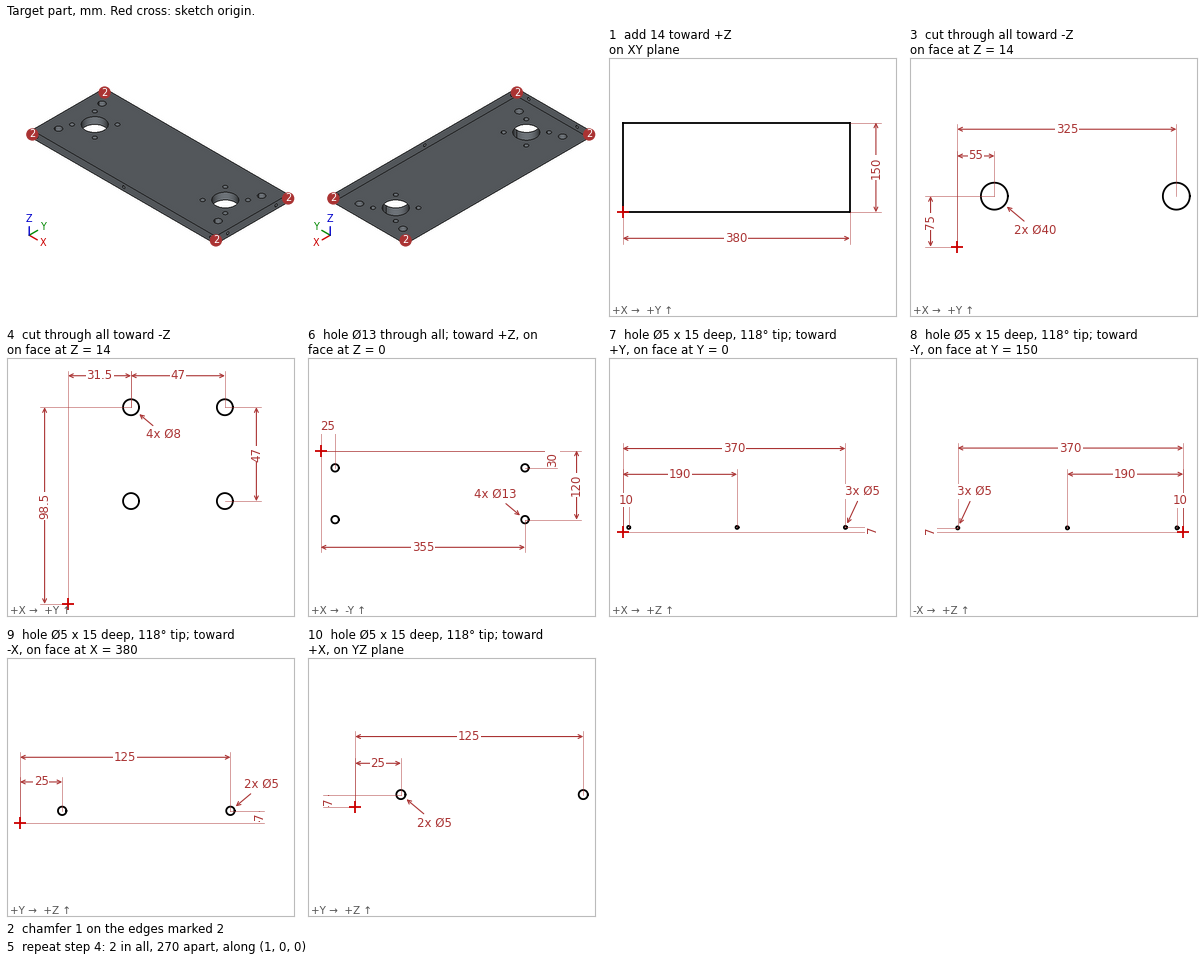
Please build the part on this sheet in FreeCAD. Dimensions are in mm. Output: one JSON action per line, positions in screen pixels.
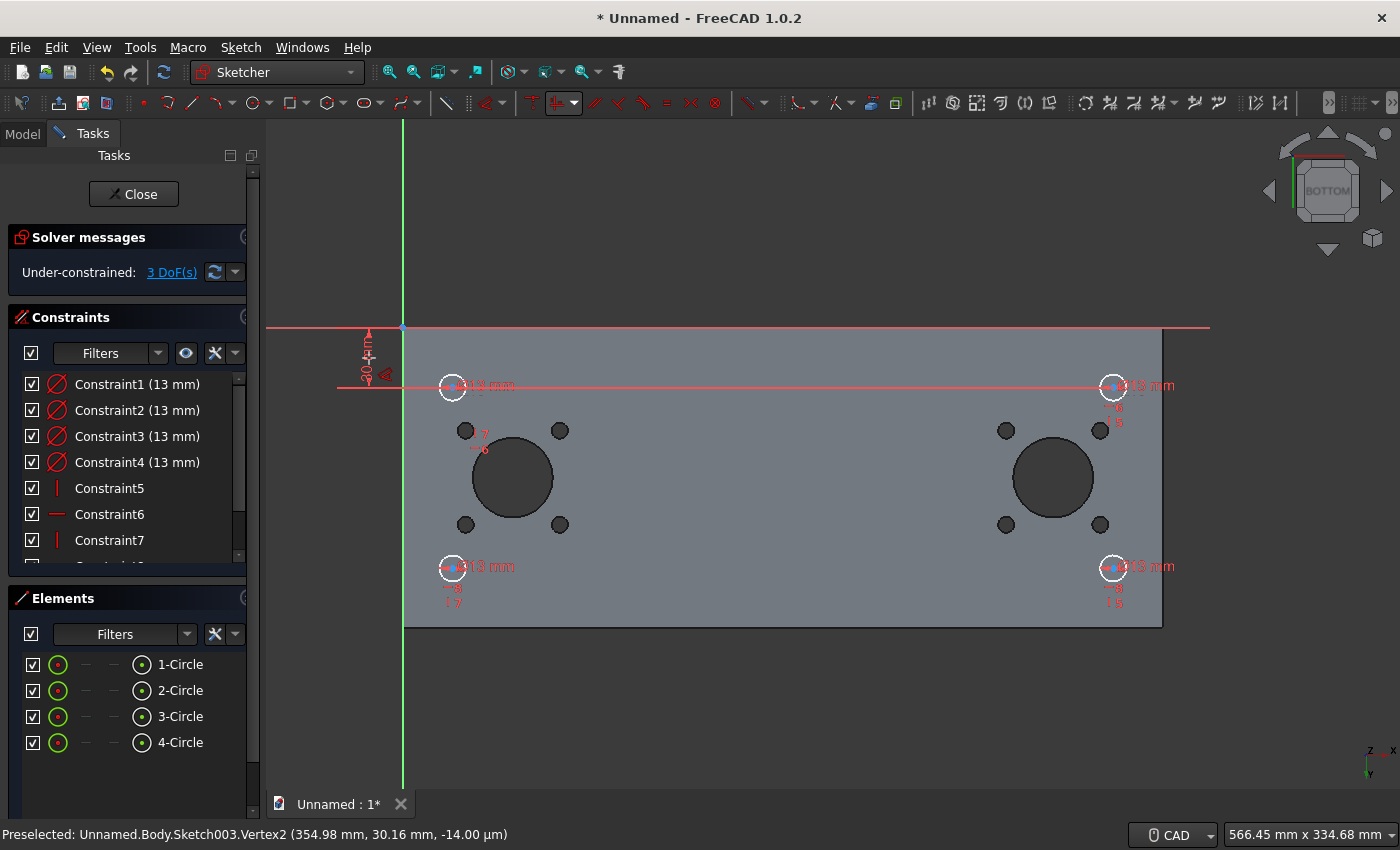
{"action": "left_click", "coordinate": [453, 388]}
{"action": "left_click", "coordinate": [428, 294]}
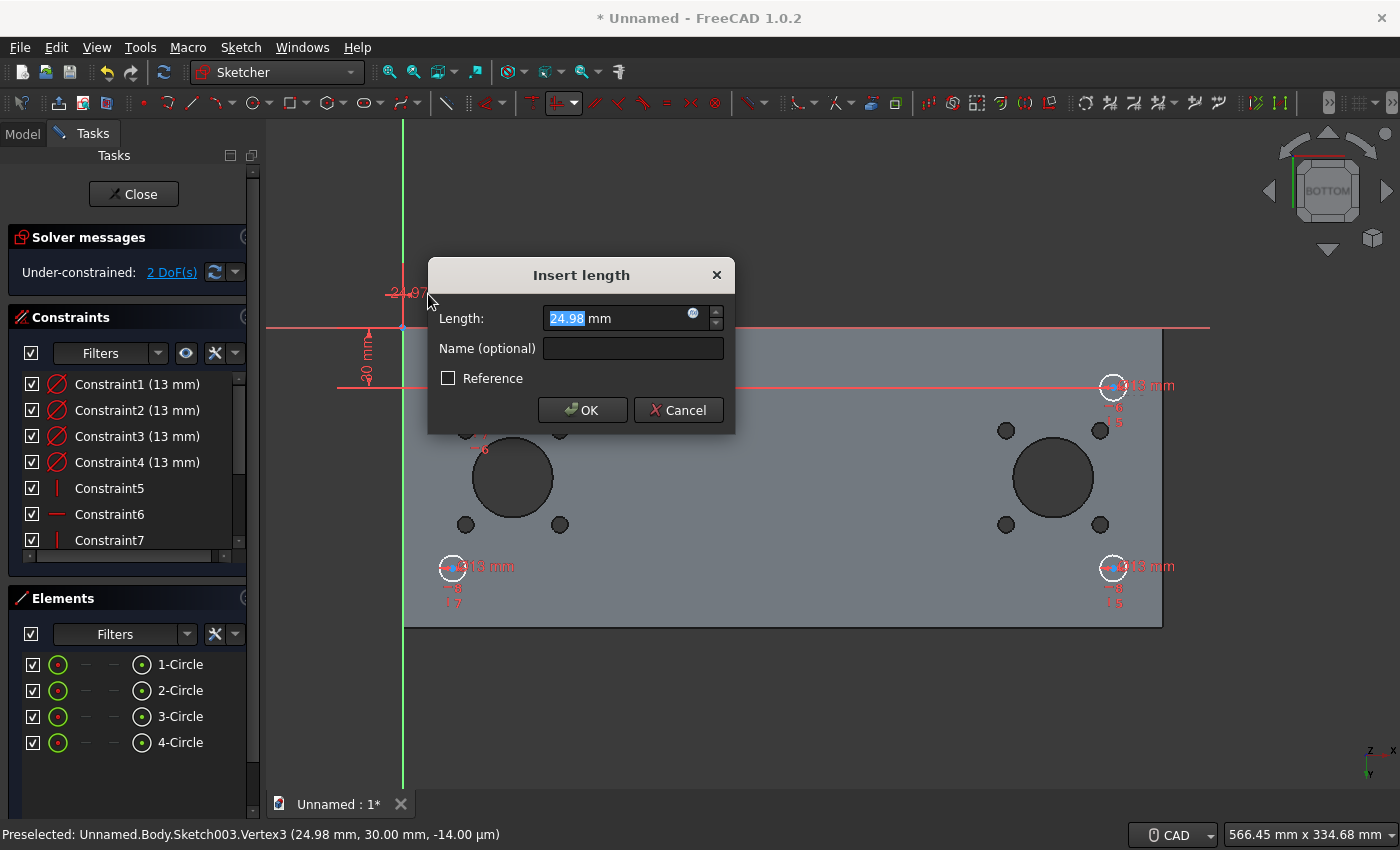
{"action": "type", "text": "25"}
{"action": "key", "text": "Return"}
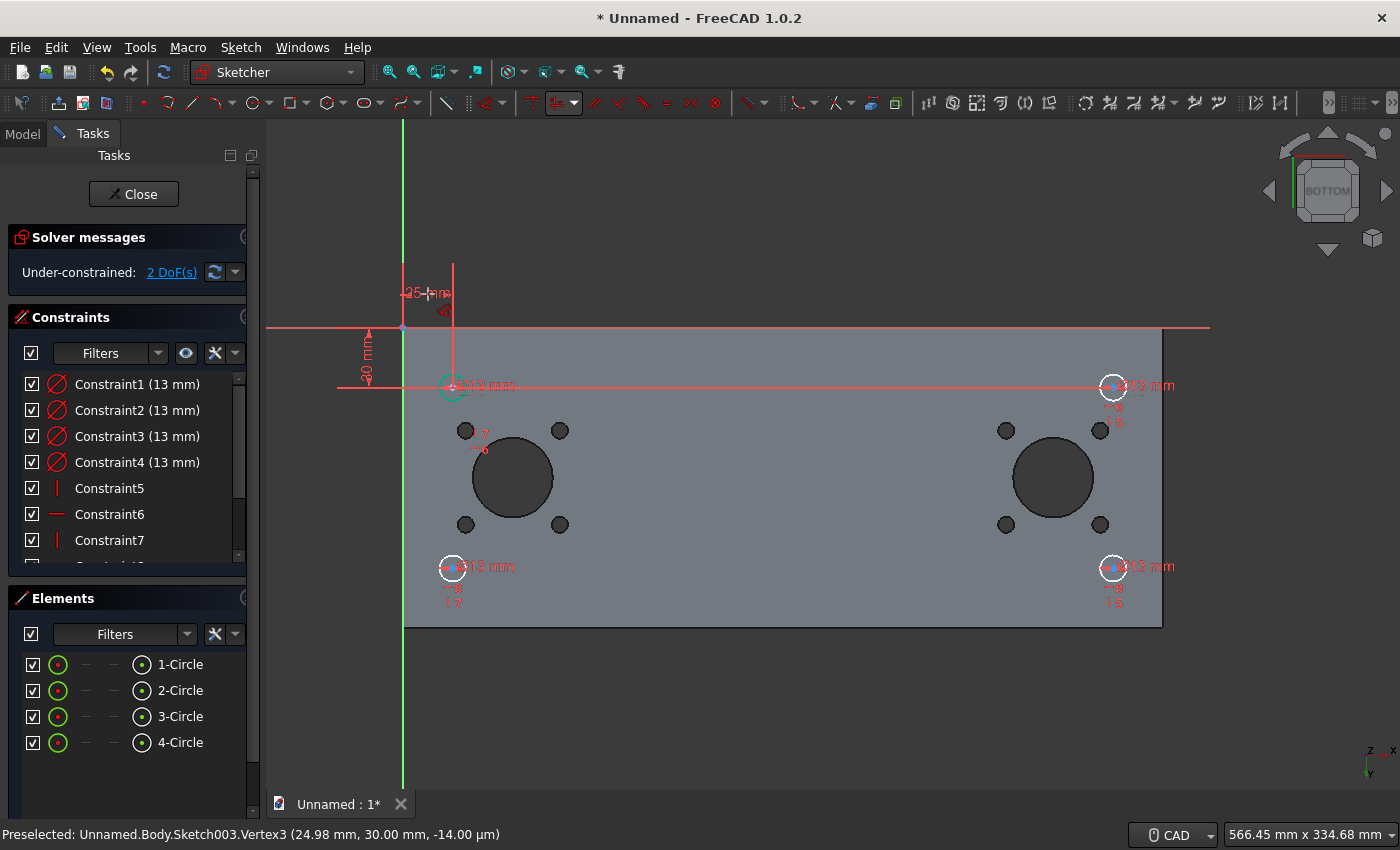
{"action": "left_click", "coordinate": [1113, 568]}
{"action": "left_click", "coordinate": [758, 294]}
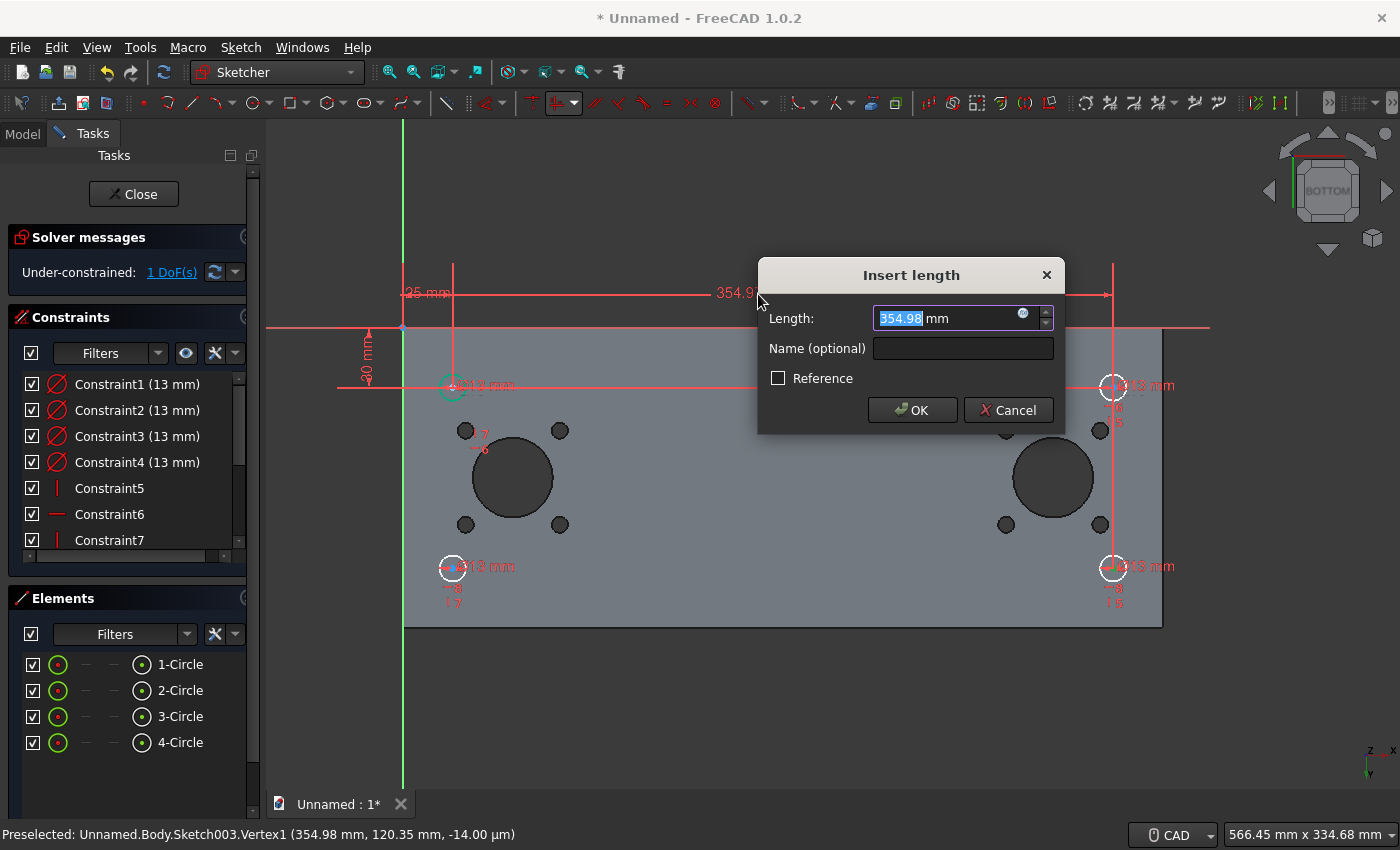
{"action": "type", "text": "355"}
{"action": "key", "text": "Return"}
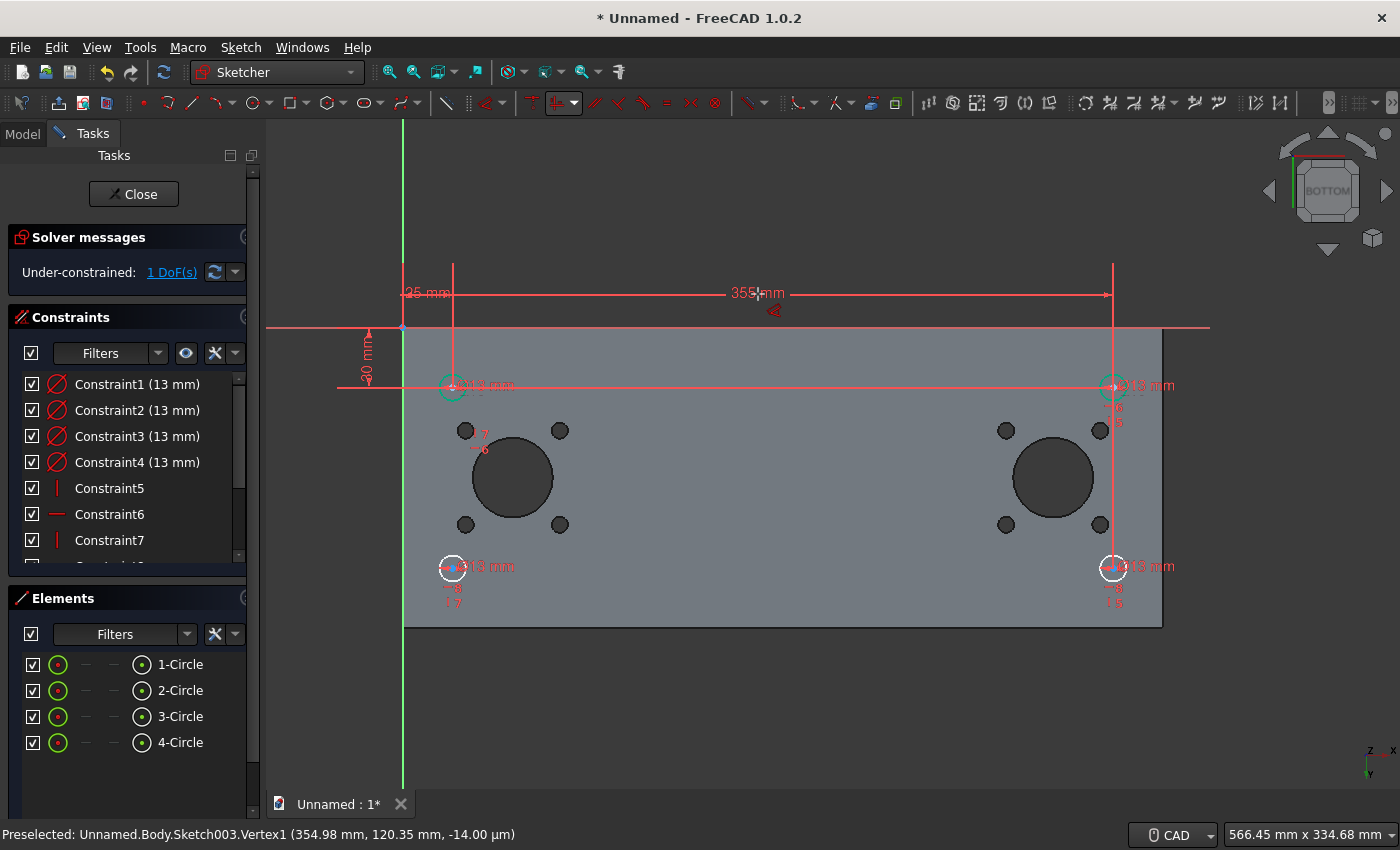
{"action": "left_click", "coordinate": [1113, 568]}
{"action": "left_click", "coordinate": [369, 448]}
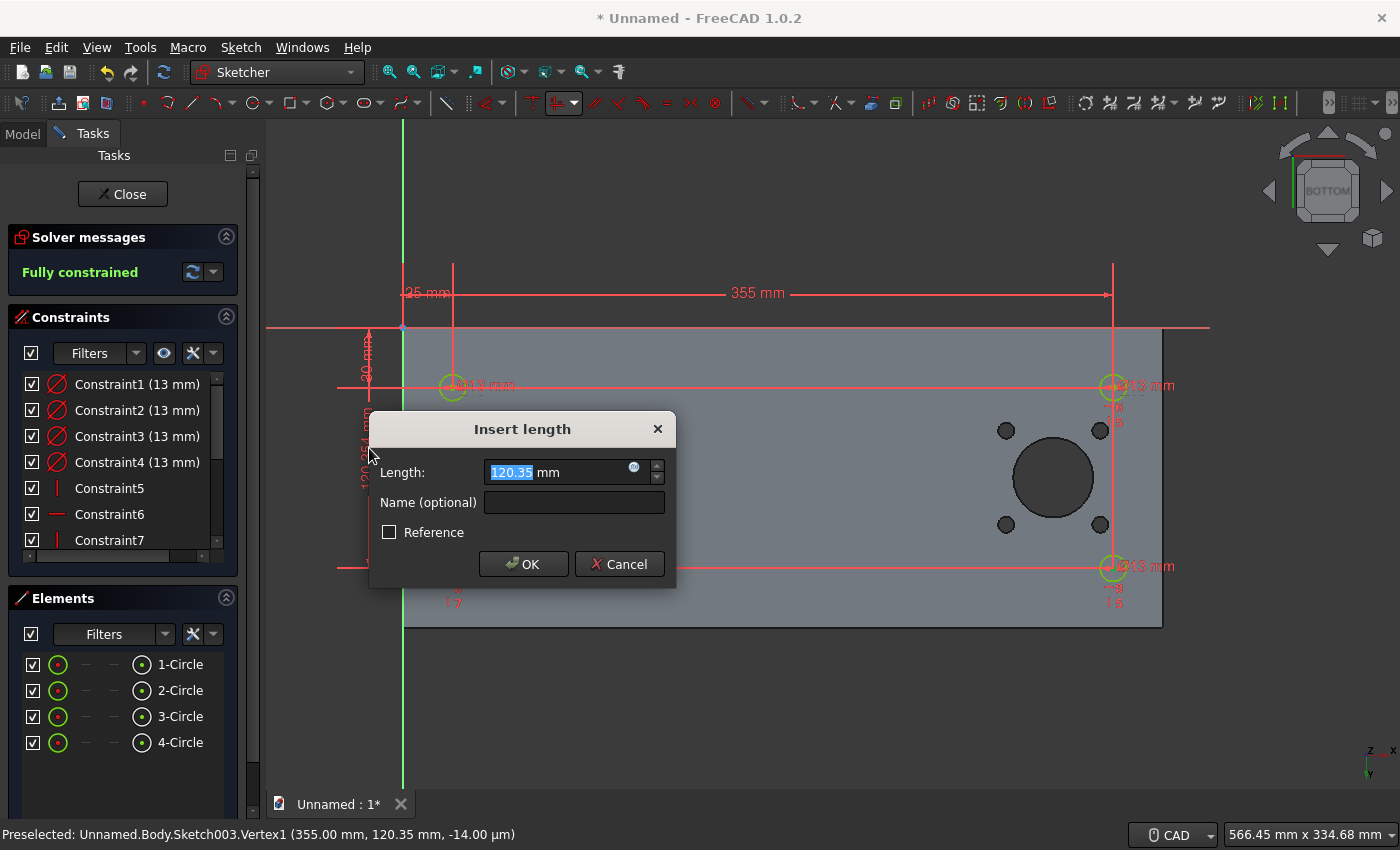
{"action": "type", "text": "120"}
{"action": "key", "text": "Return"}
{"action": "key", "text": "Escape"}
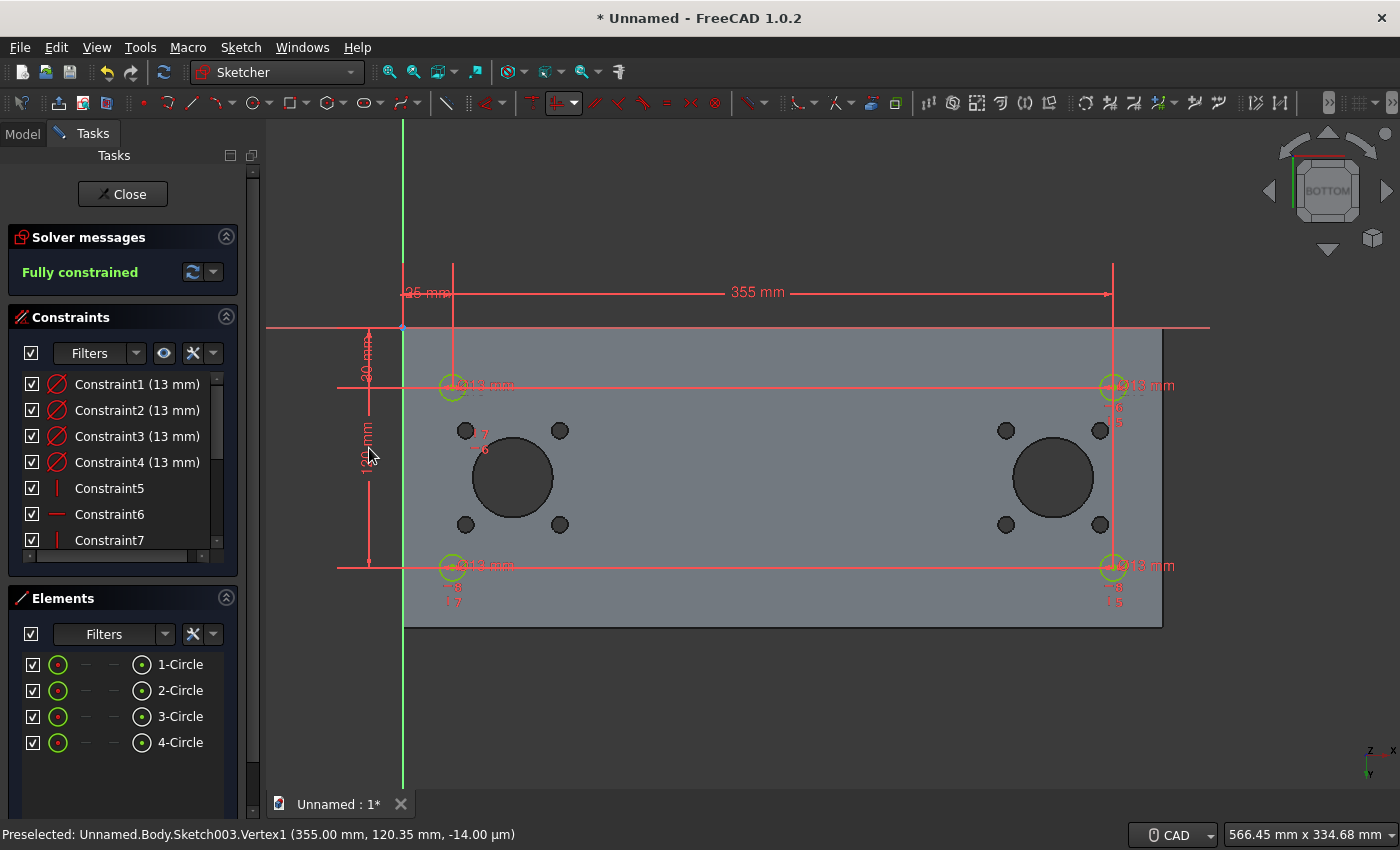
{"action": "left_click", "coordinate": [123, 194]}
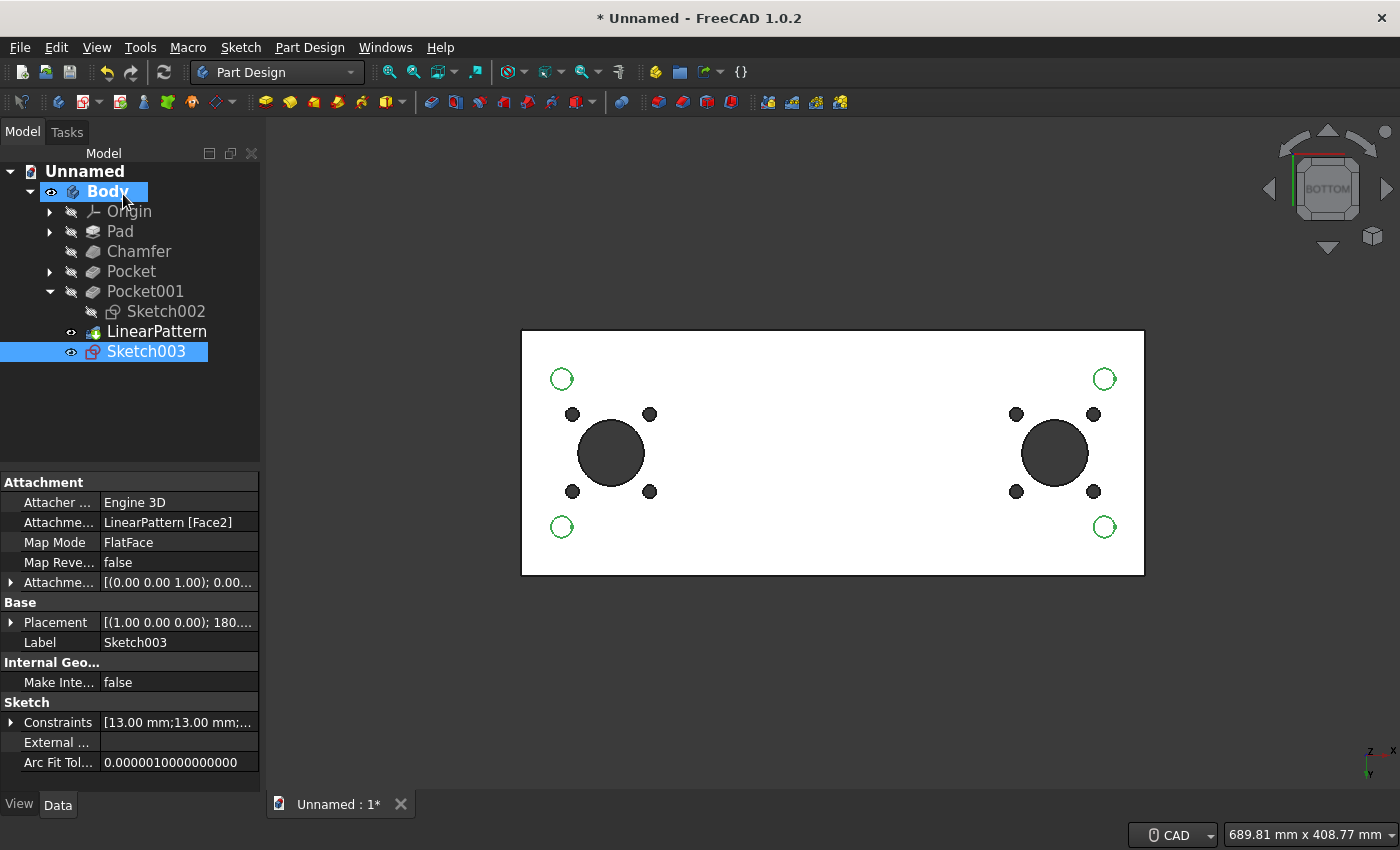
{"action": "left_click", "coordinate": [456, 102]}